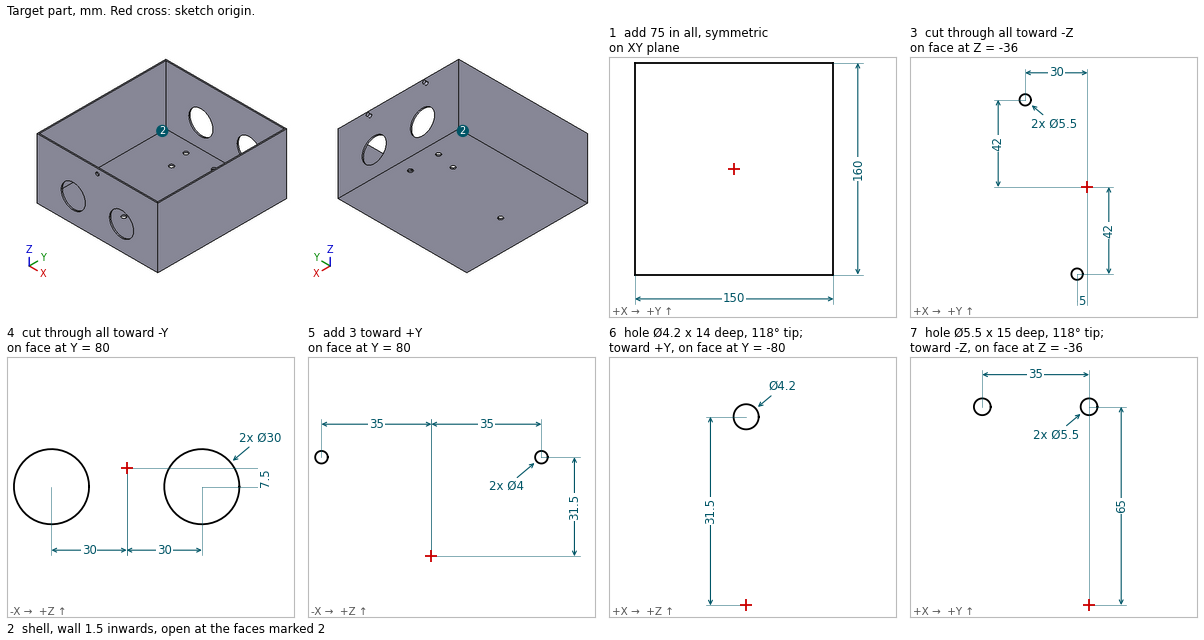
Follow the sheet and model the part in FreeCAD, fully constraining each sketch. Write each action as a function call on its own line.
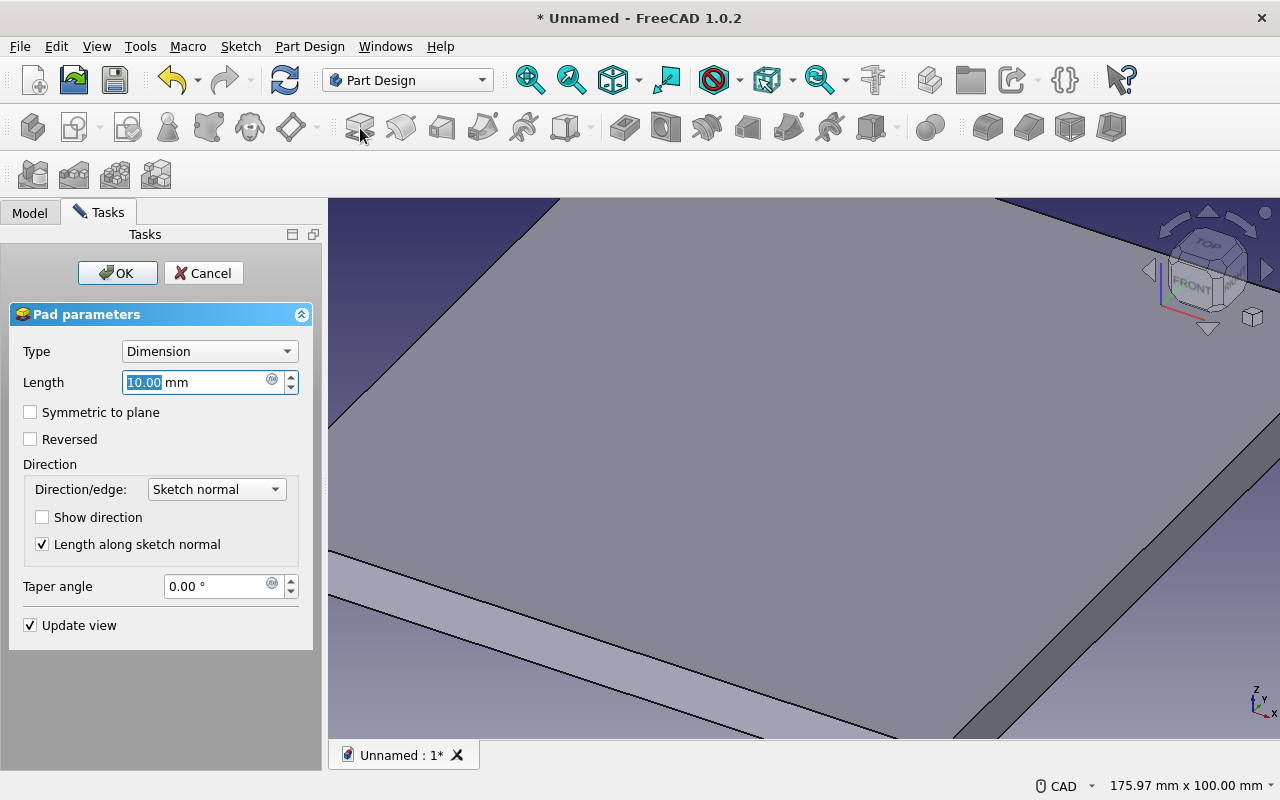
text(75)
key(Tab)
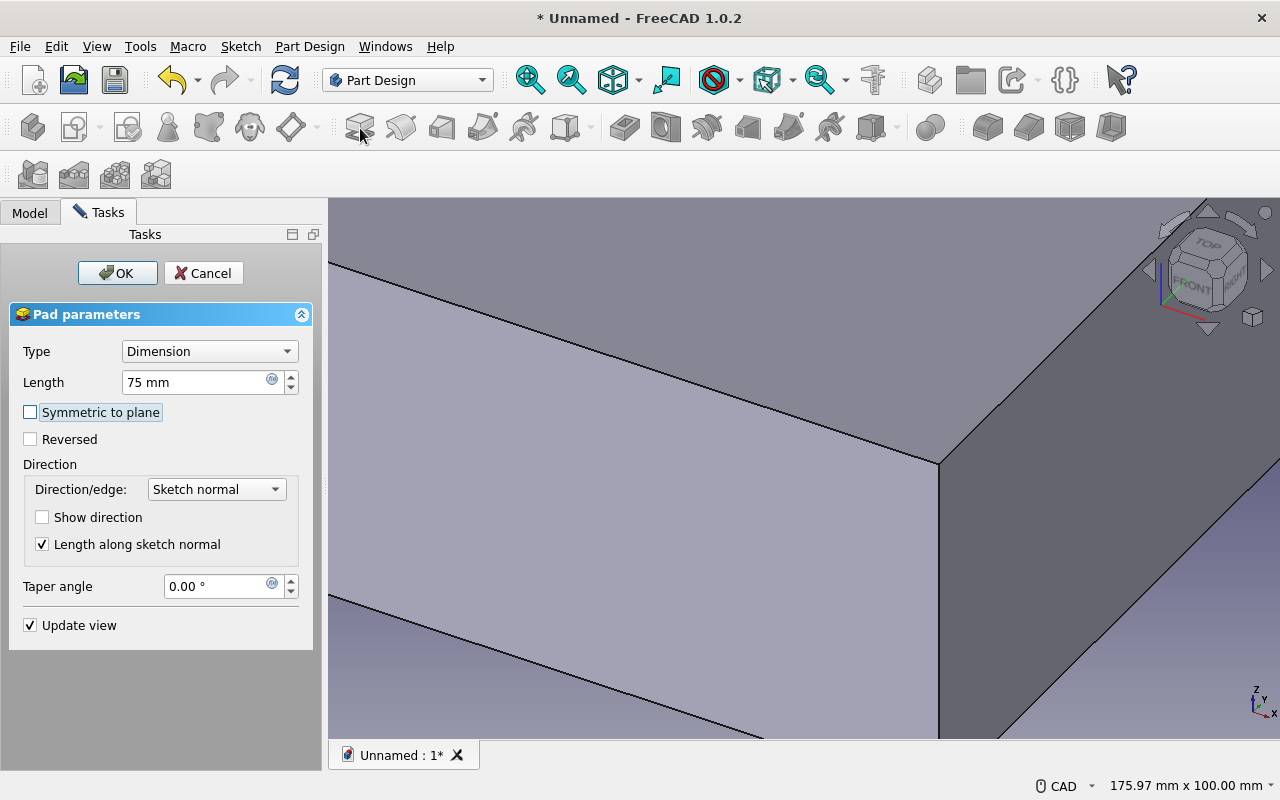
click(31, 412)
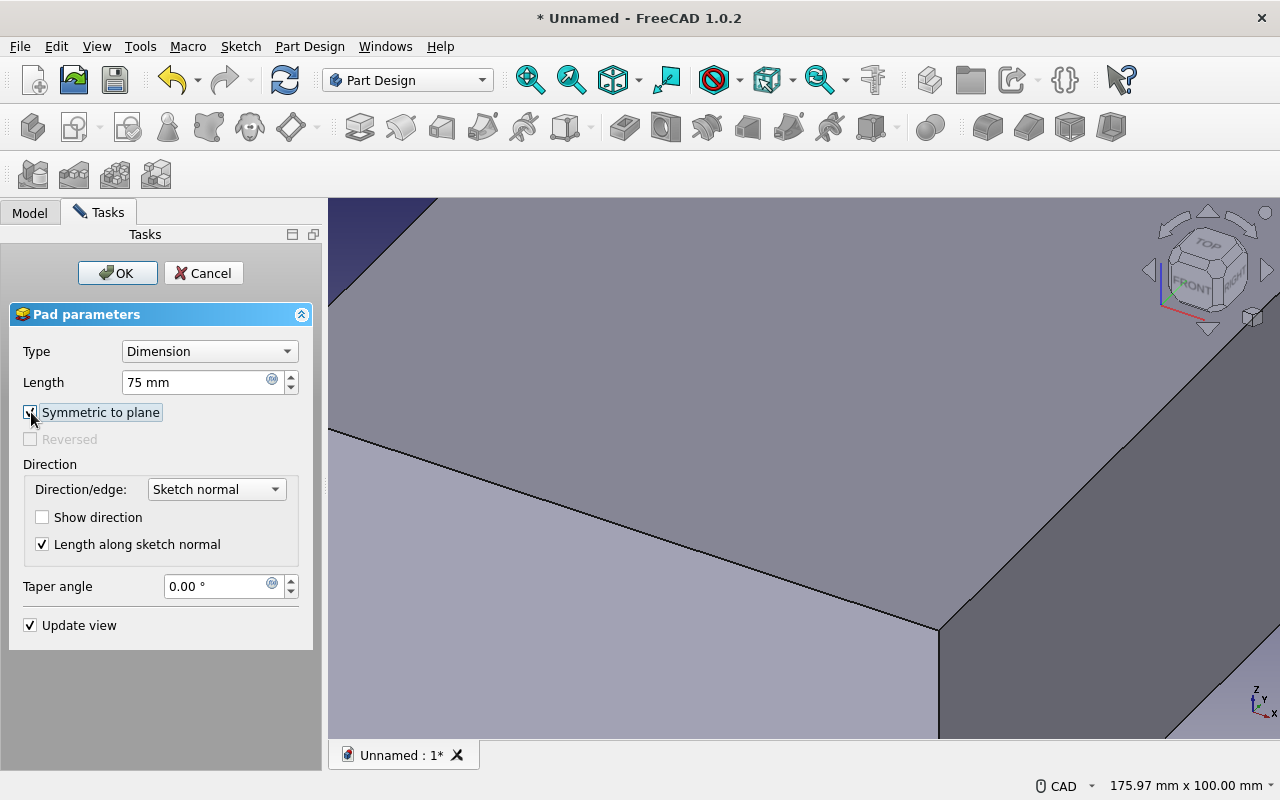
click(118, 273)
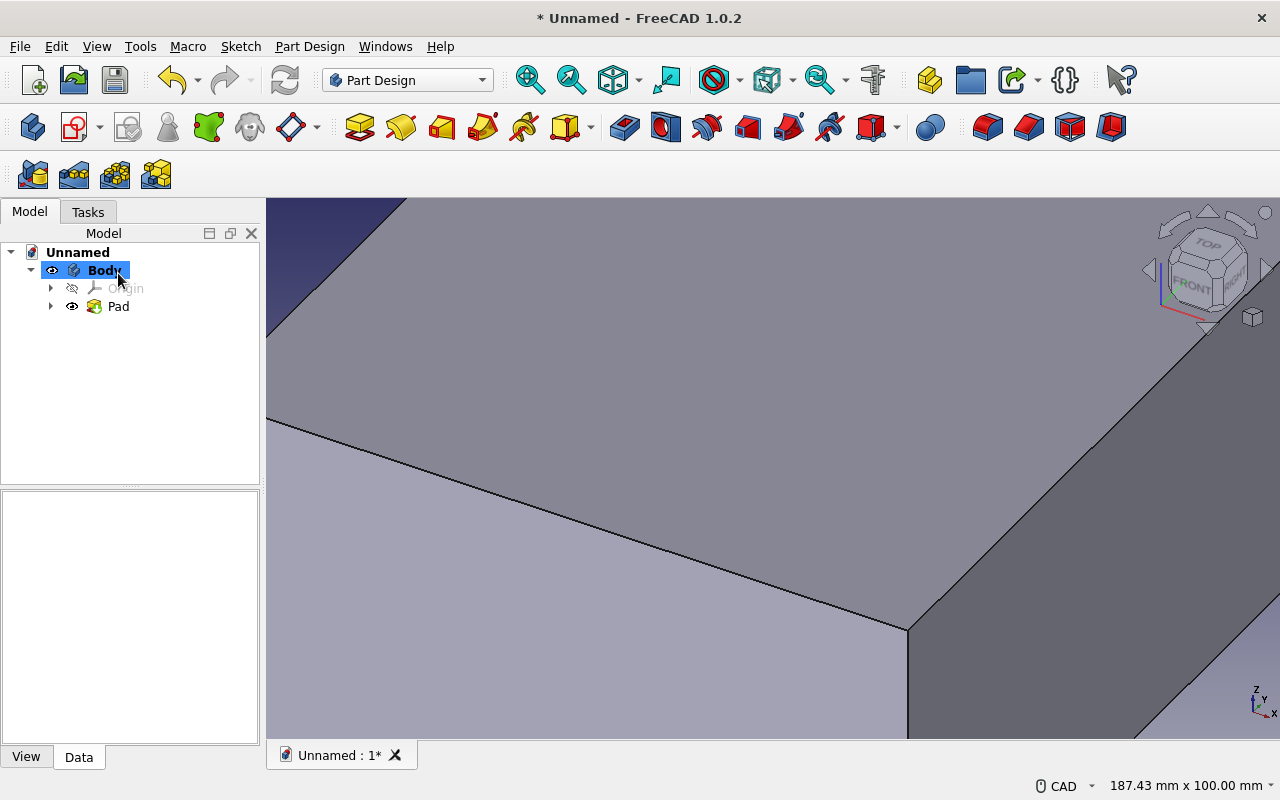
click(531, 80)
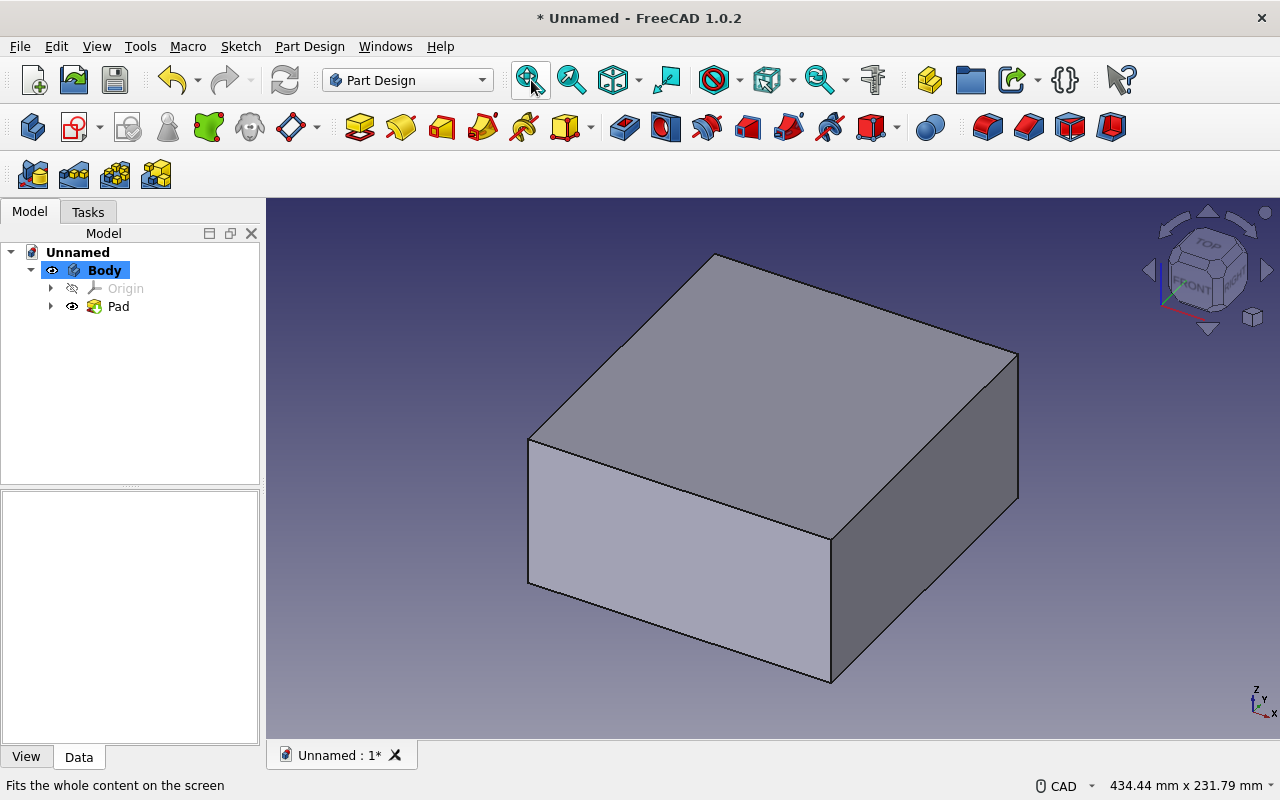
click(773, 396)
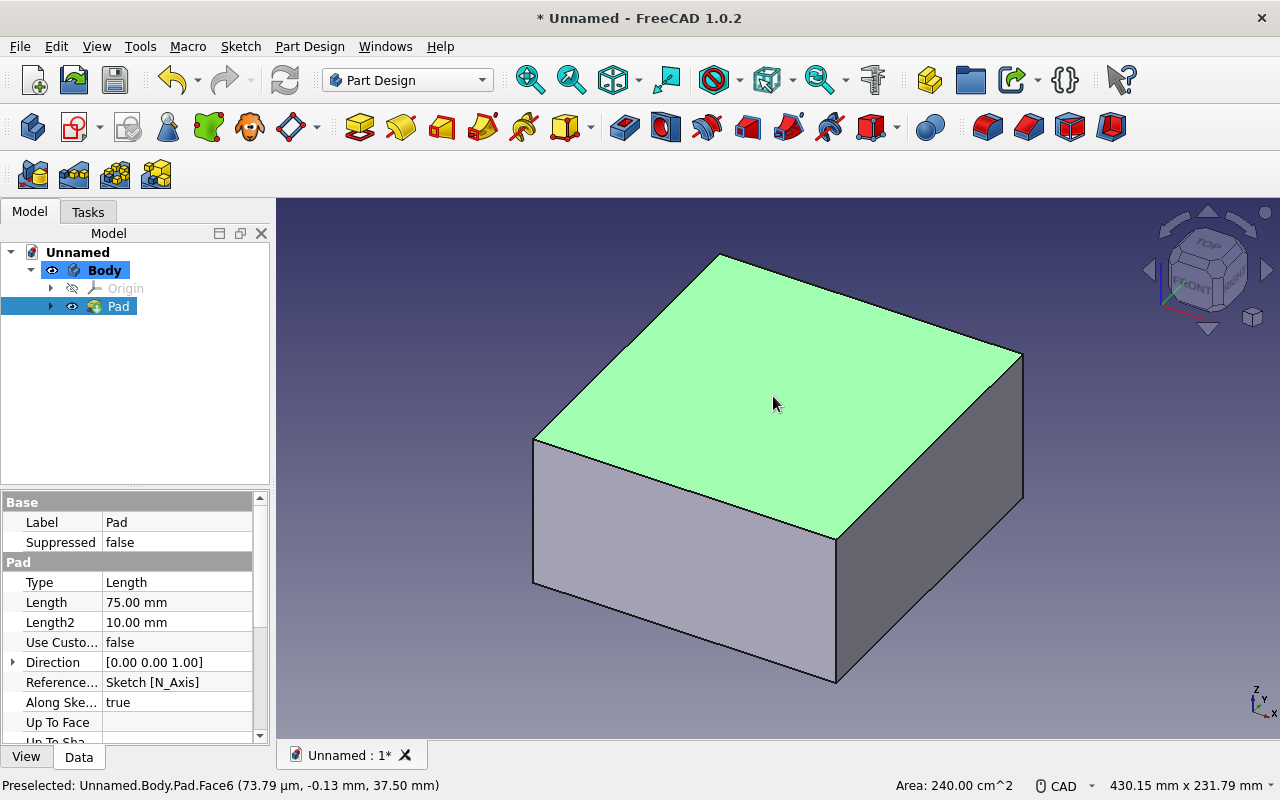
click(1111, 128)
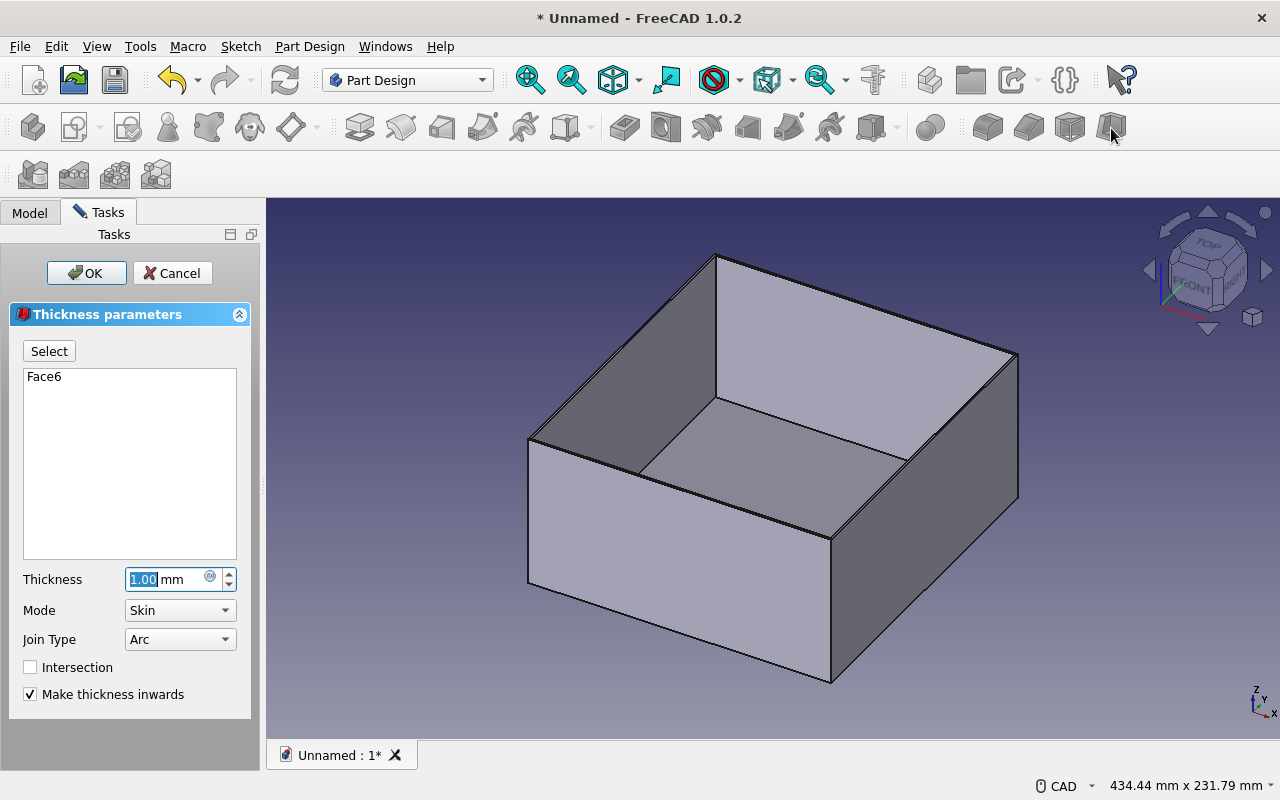
text(1.5)
key(Tab)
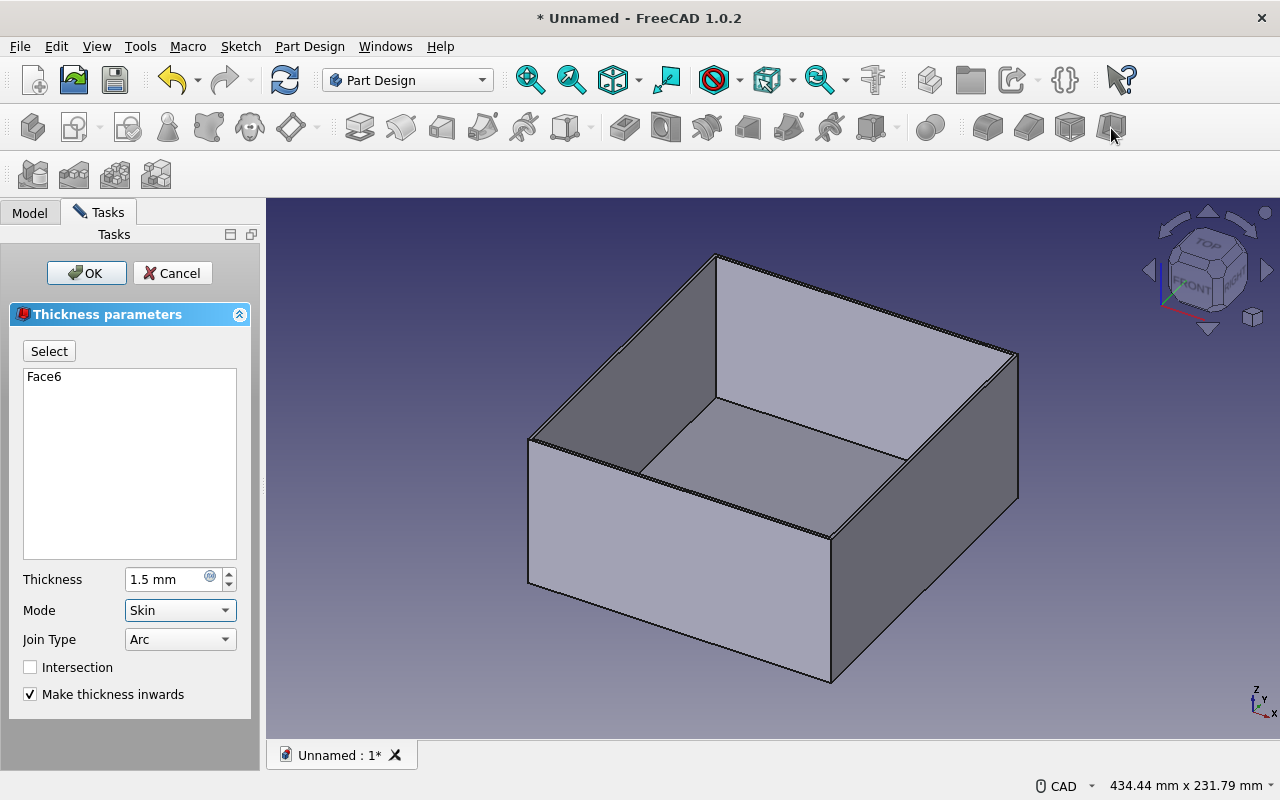
click(181, 640)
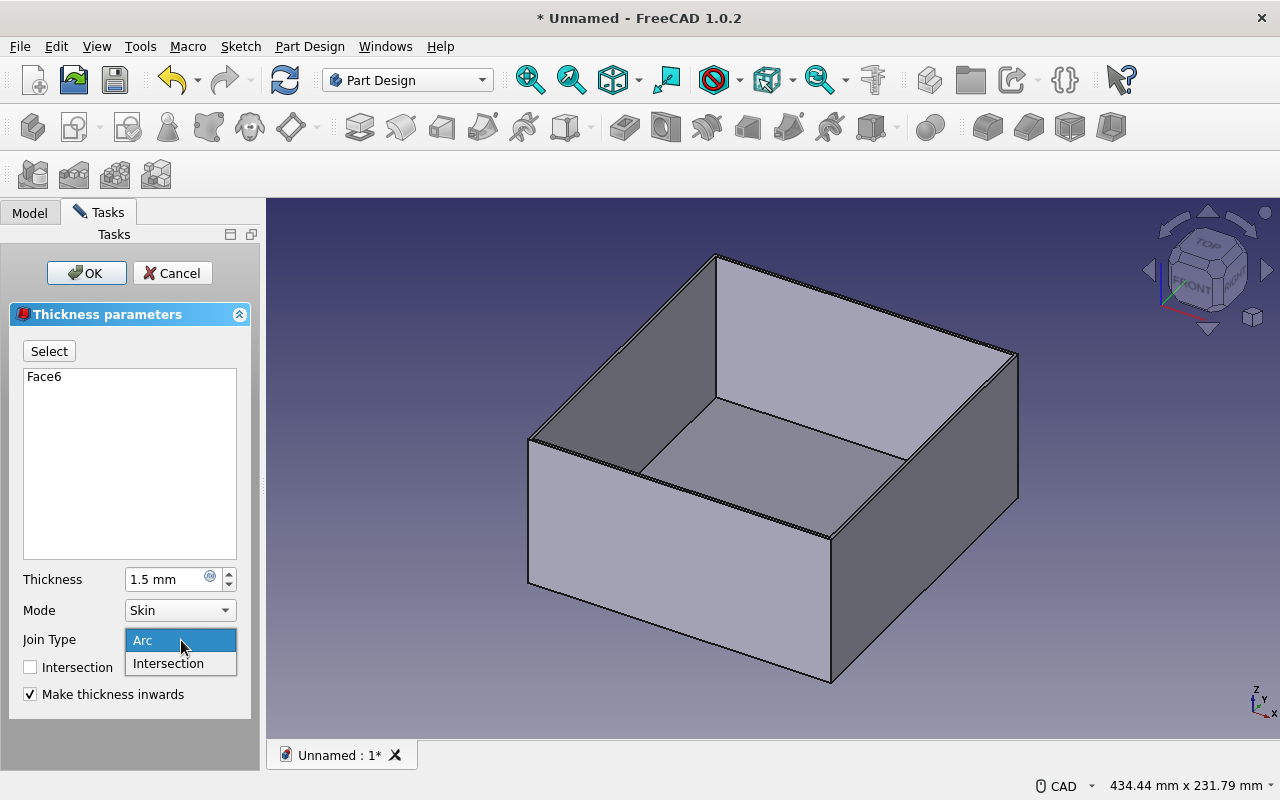
click(179, 664)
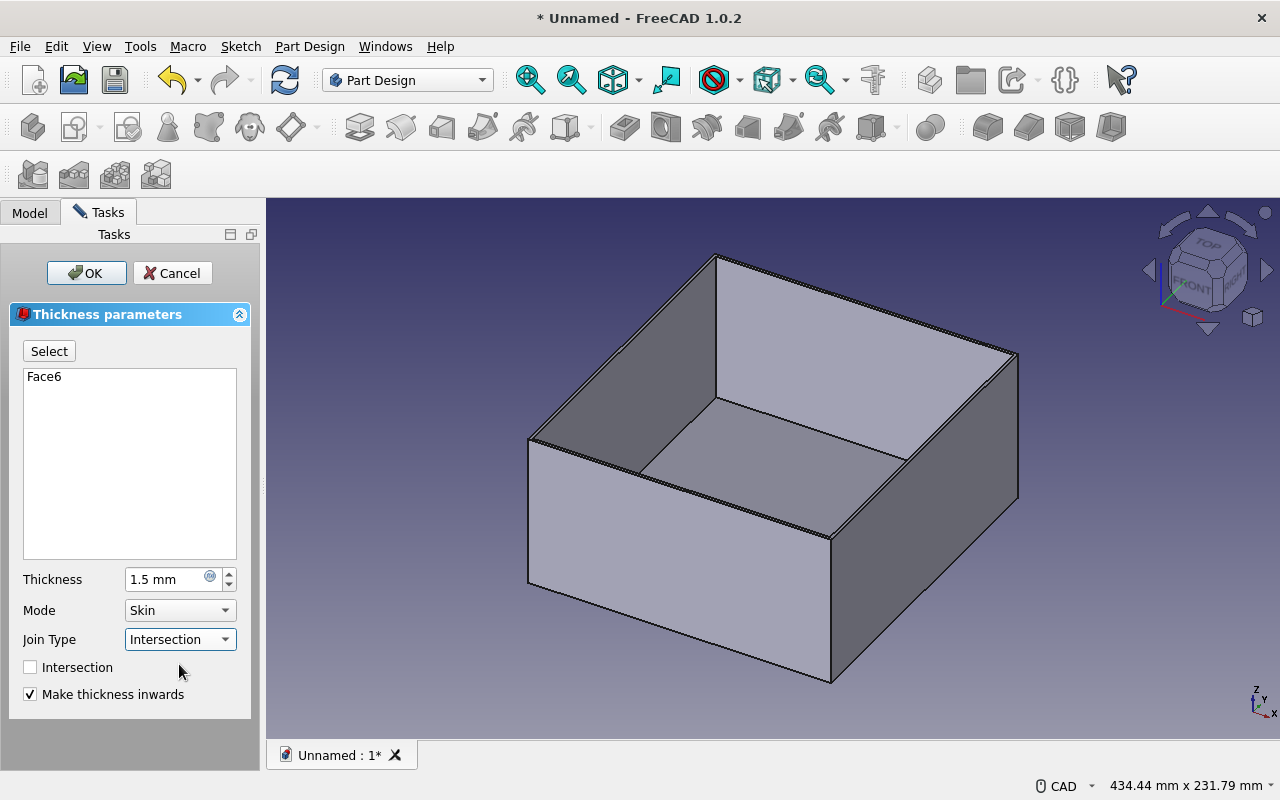
click(87, 273)